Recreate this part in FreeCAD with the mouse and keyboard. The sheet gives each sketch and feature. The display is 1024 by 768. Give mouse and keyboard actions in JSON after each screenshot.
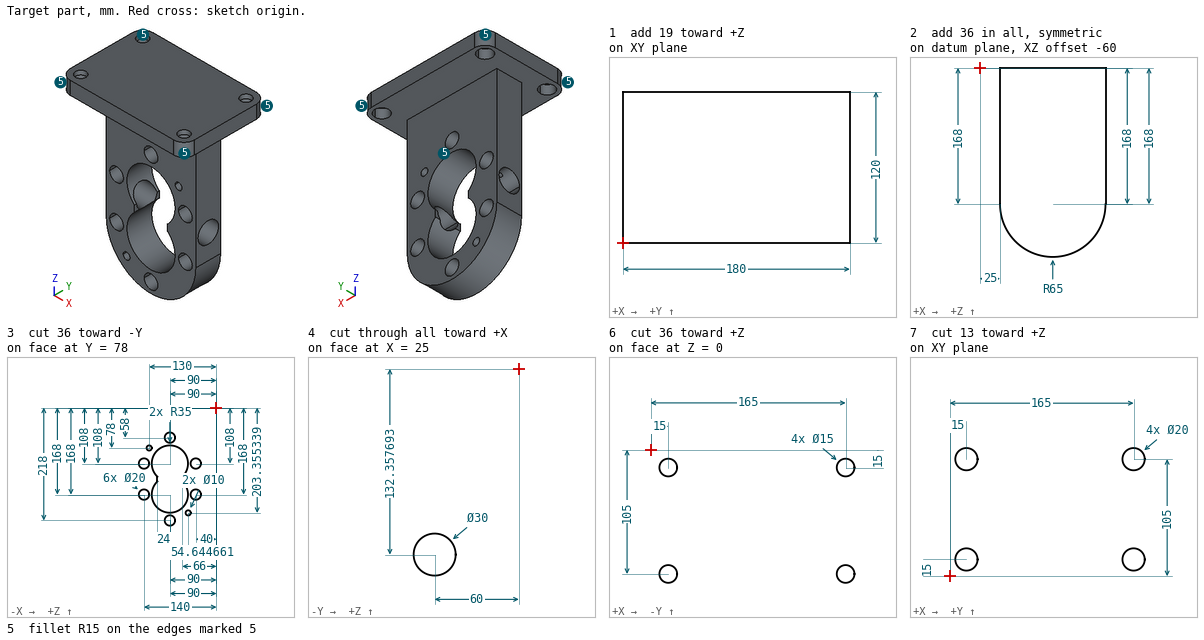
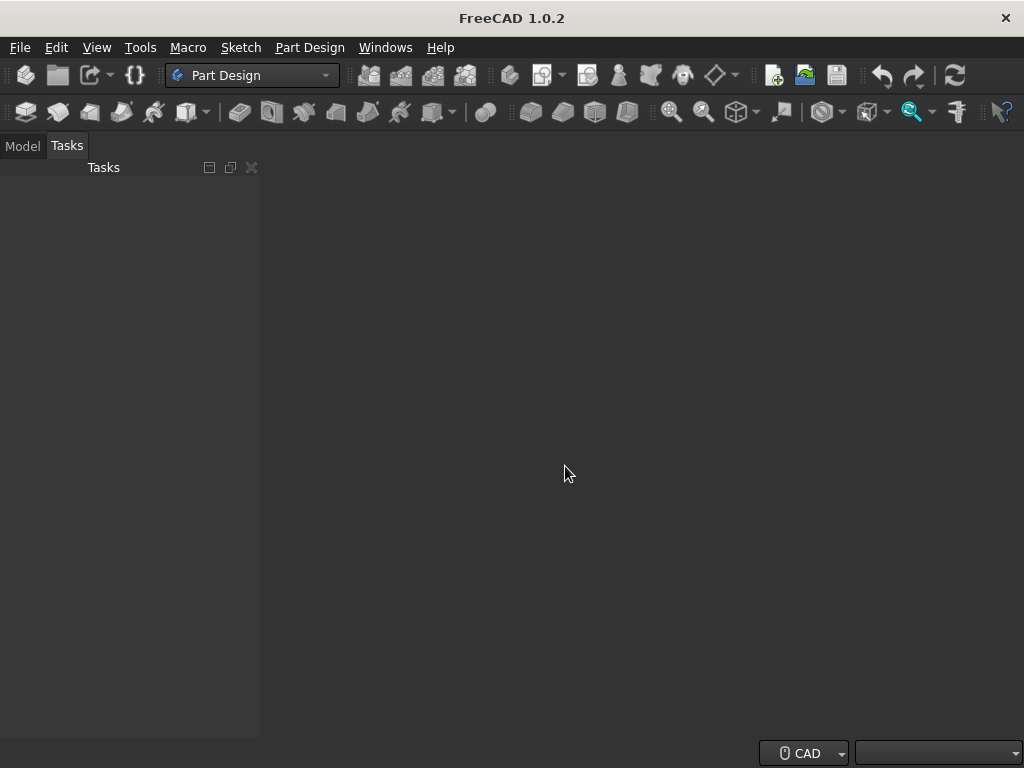
{"action": "left_click", "coordinate": [774, 76]}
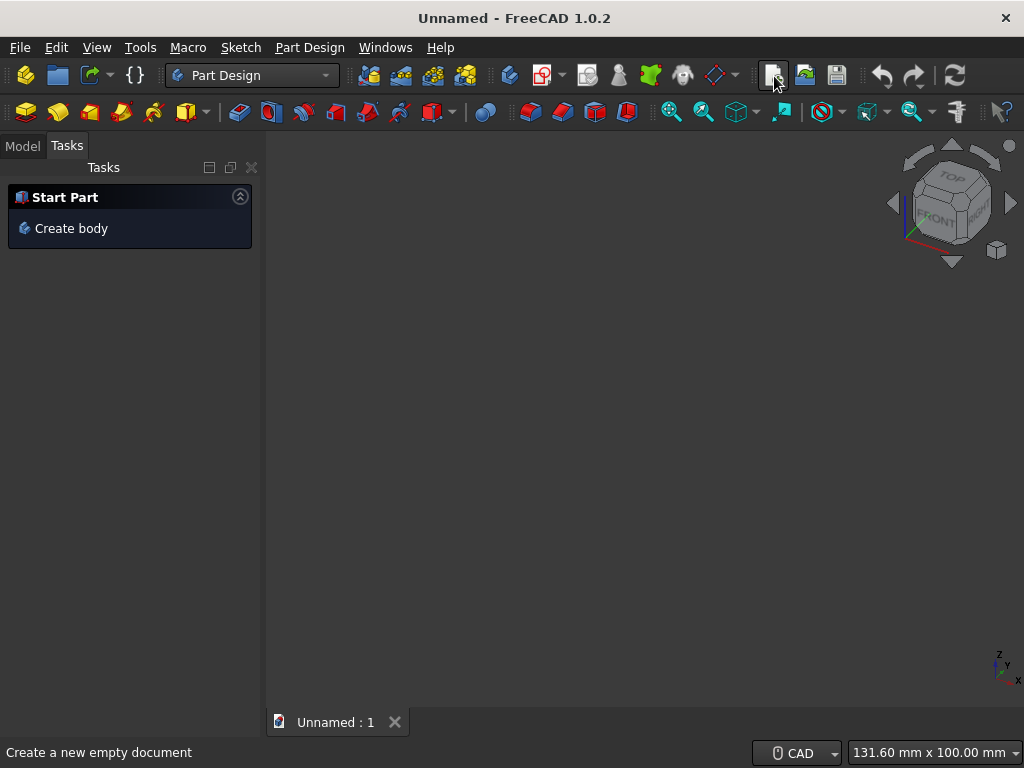
{"action": "left_click", "coordinate": [542, 76]}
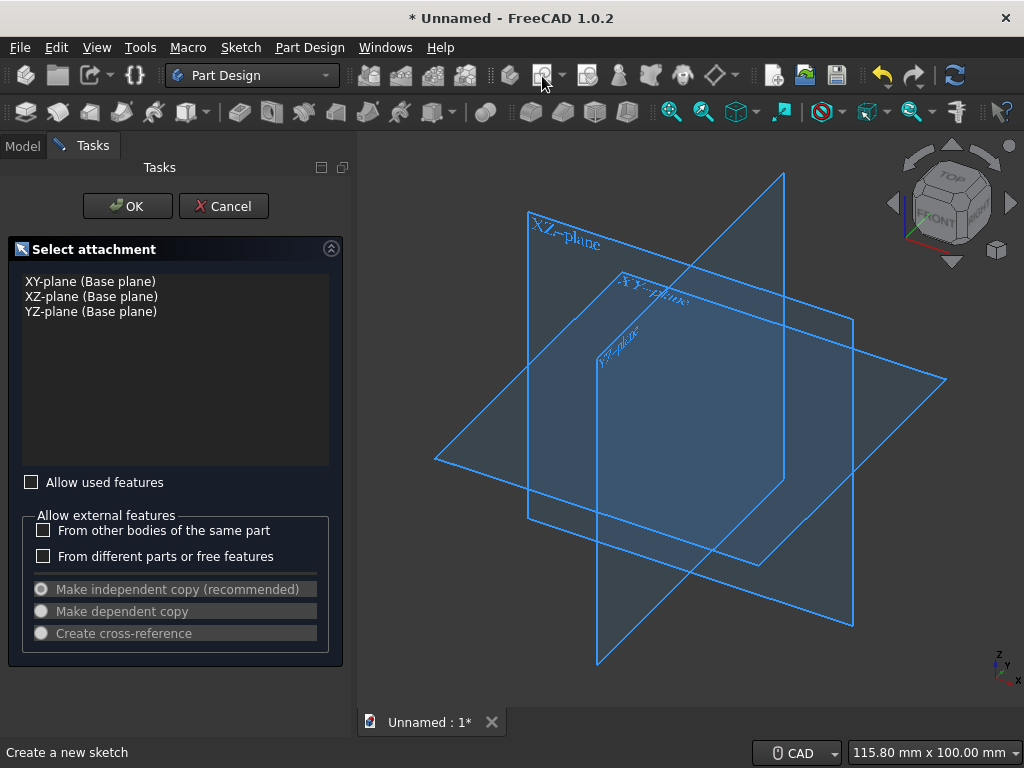
{"action": "left_click", "coordinate": [82, 282]}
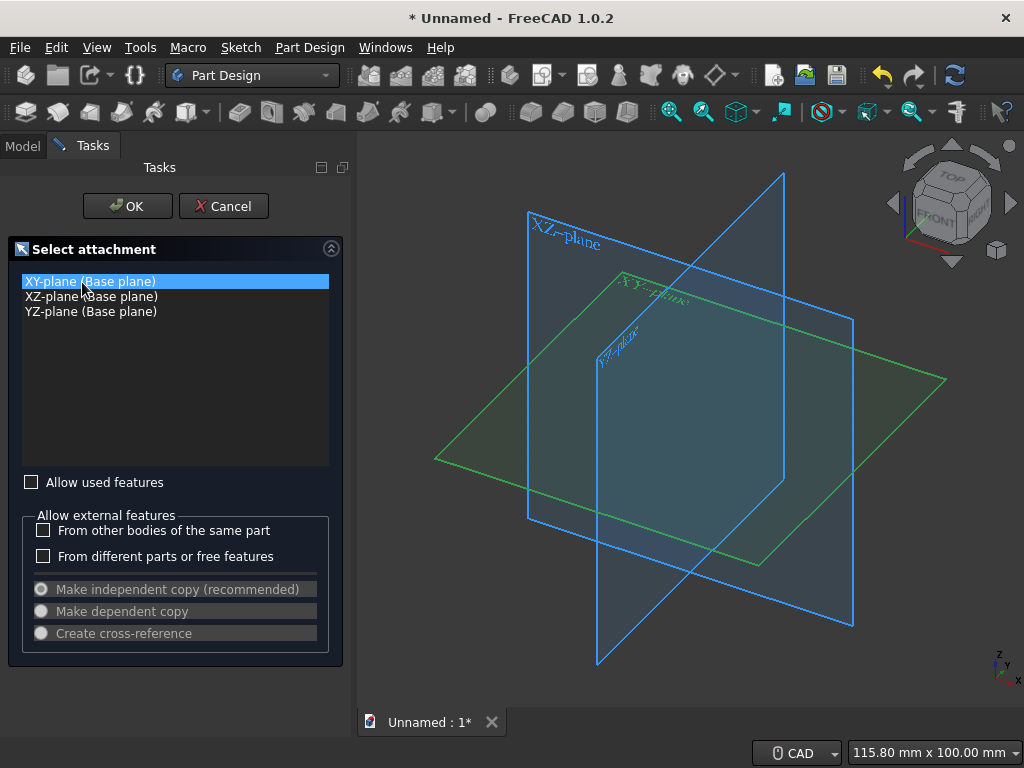
{"action": "left_click", "coordinate": [128, 206]}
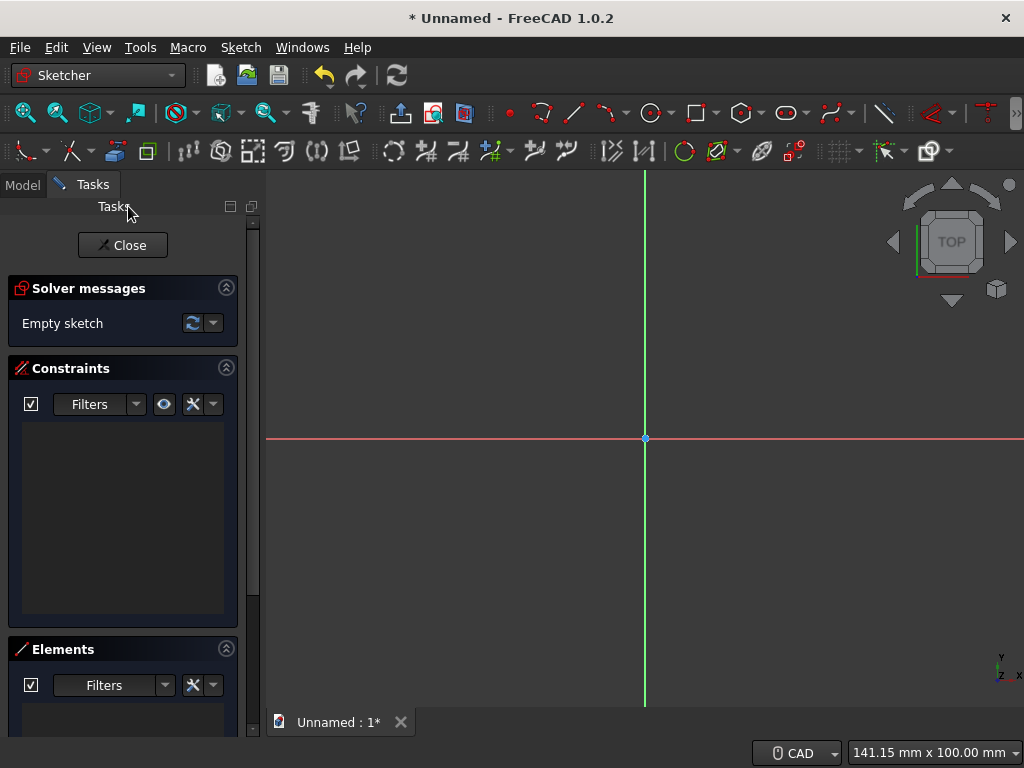
{"action": "scroll", "coordinate": [294, 626], "scroll_direction": "down", "scroll_amount": 5}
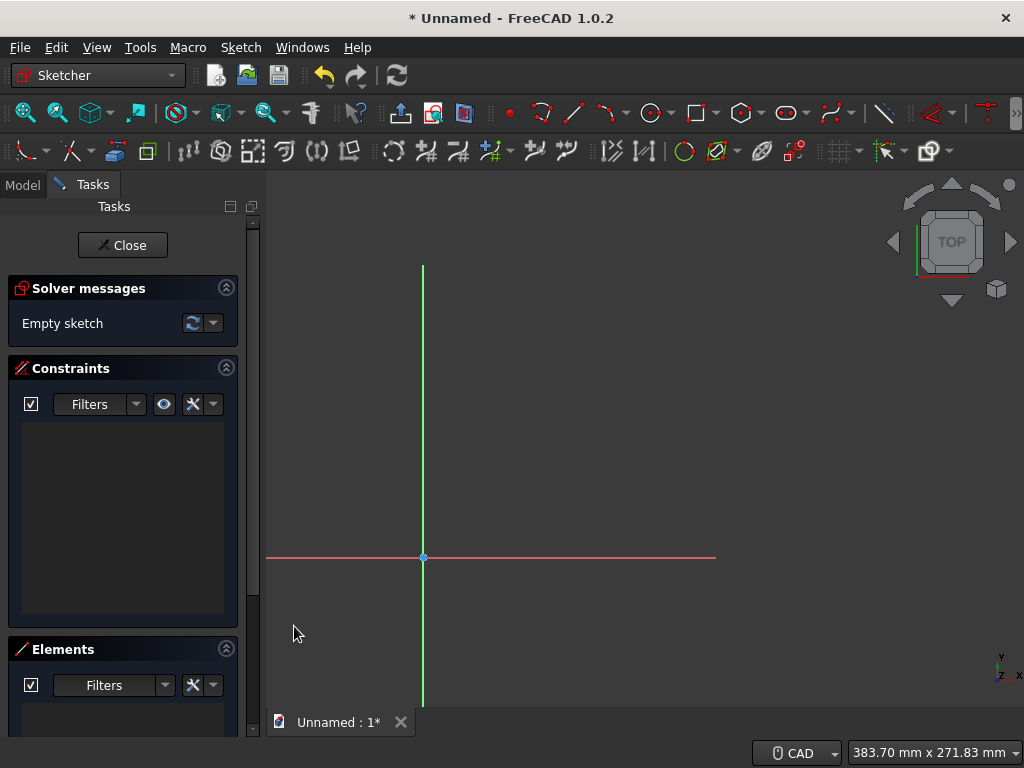
{"action": "left_click", "coordinate": [696, 114]}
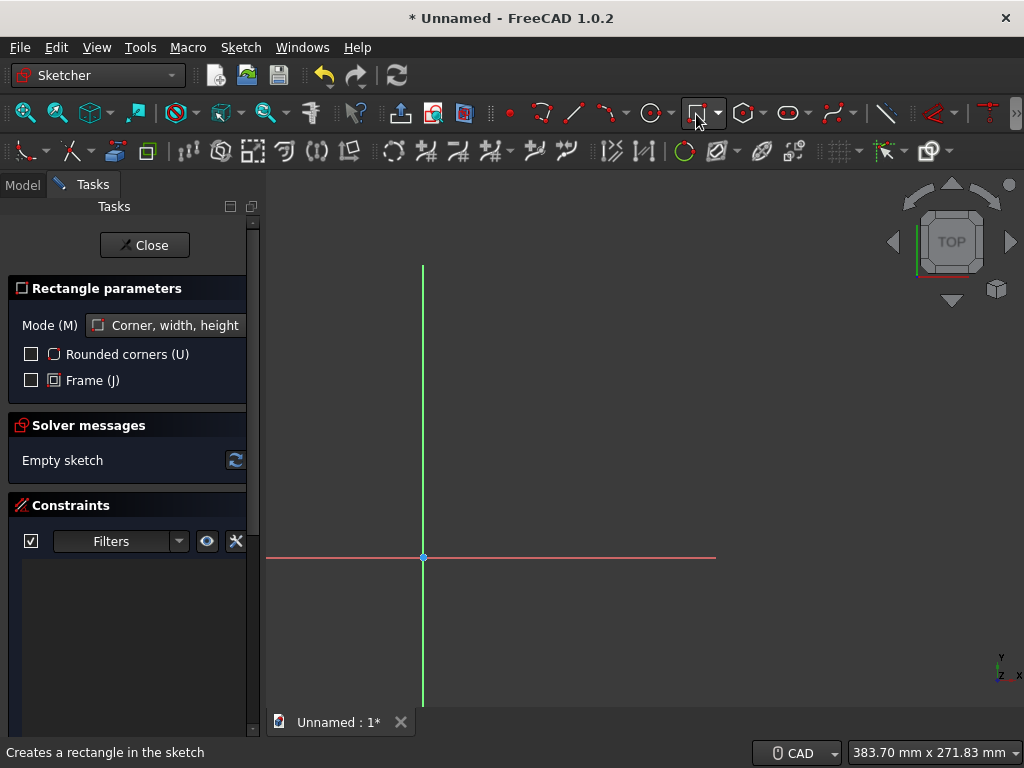
{"action": "left_click", "coordinate": [423, 558]}
{"action": "left_click", "coordinate": [779, 320]}
{"action": "key", "text": "Escape"}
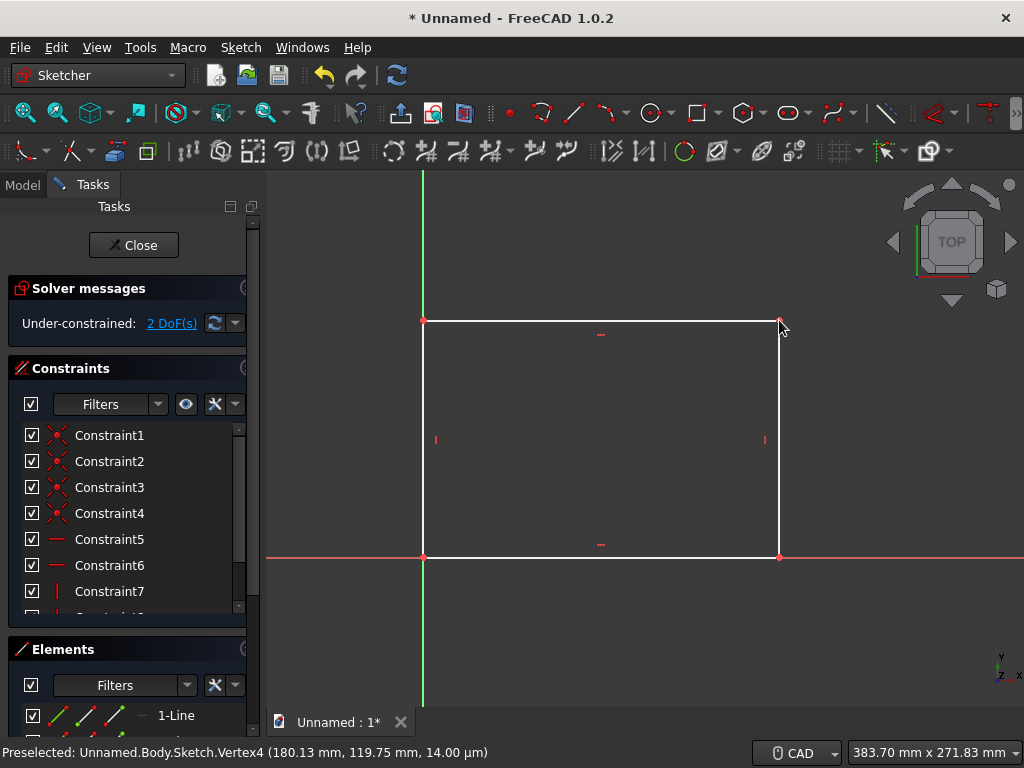
{"action": "left_click", "coordinate": [530, 558]}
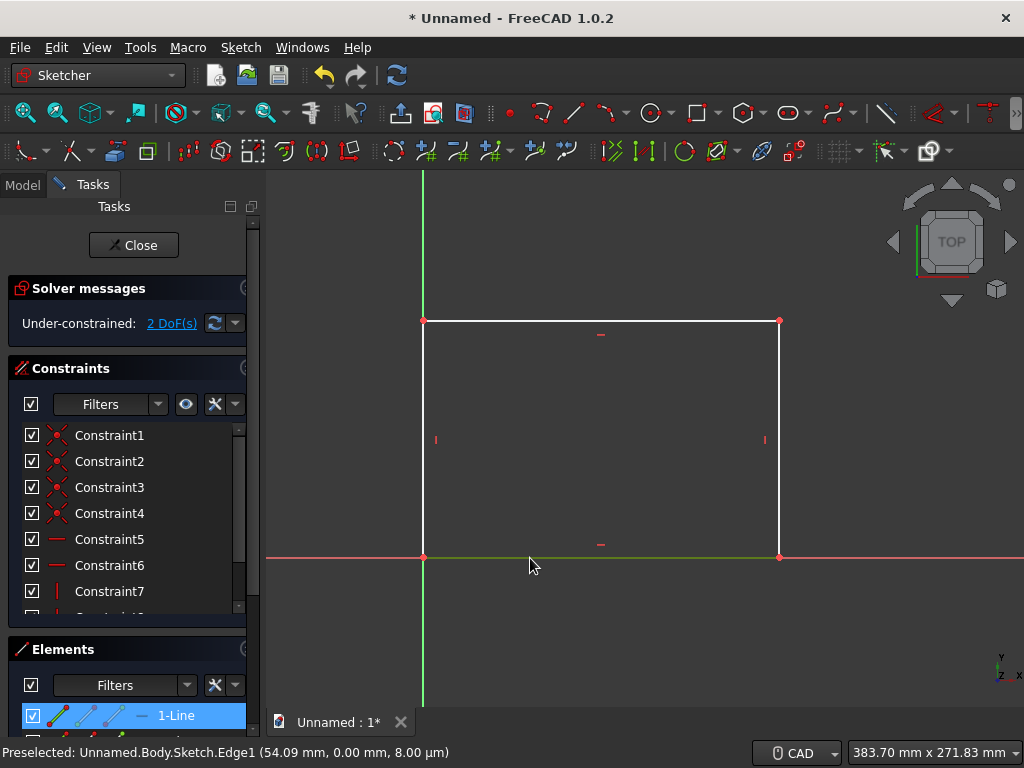
{"action": "left_click", "coordinate": [956, 114]}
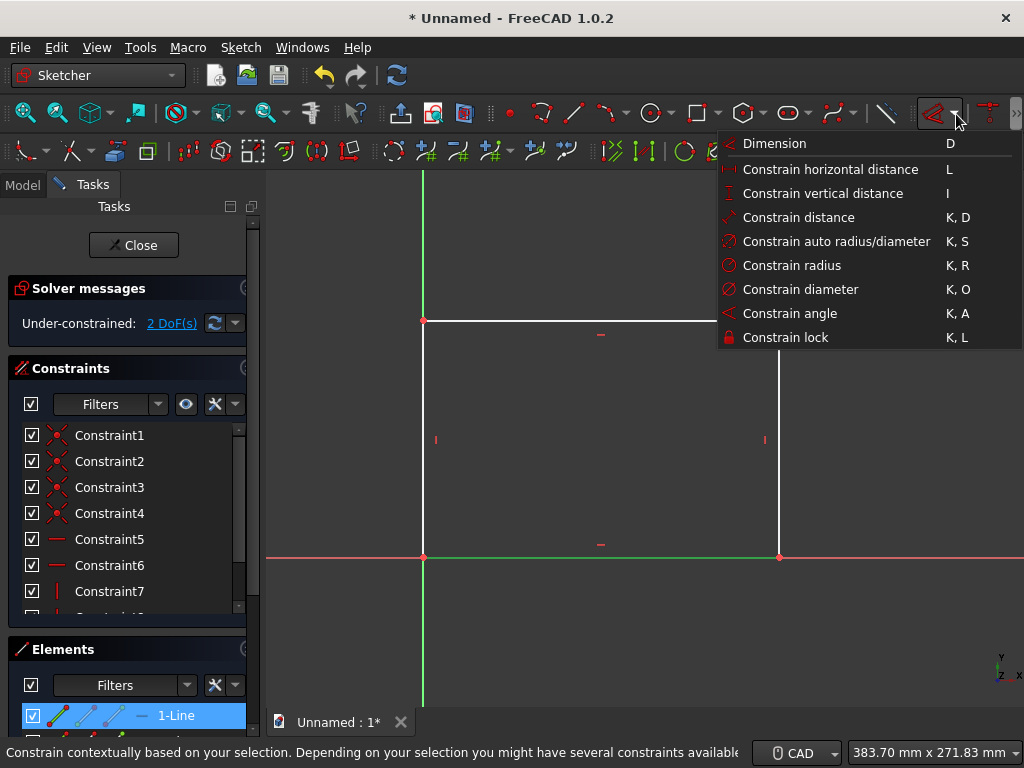
{"action": "left_click", "coordinate": [870, 169]}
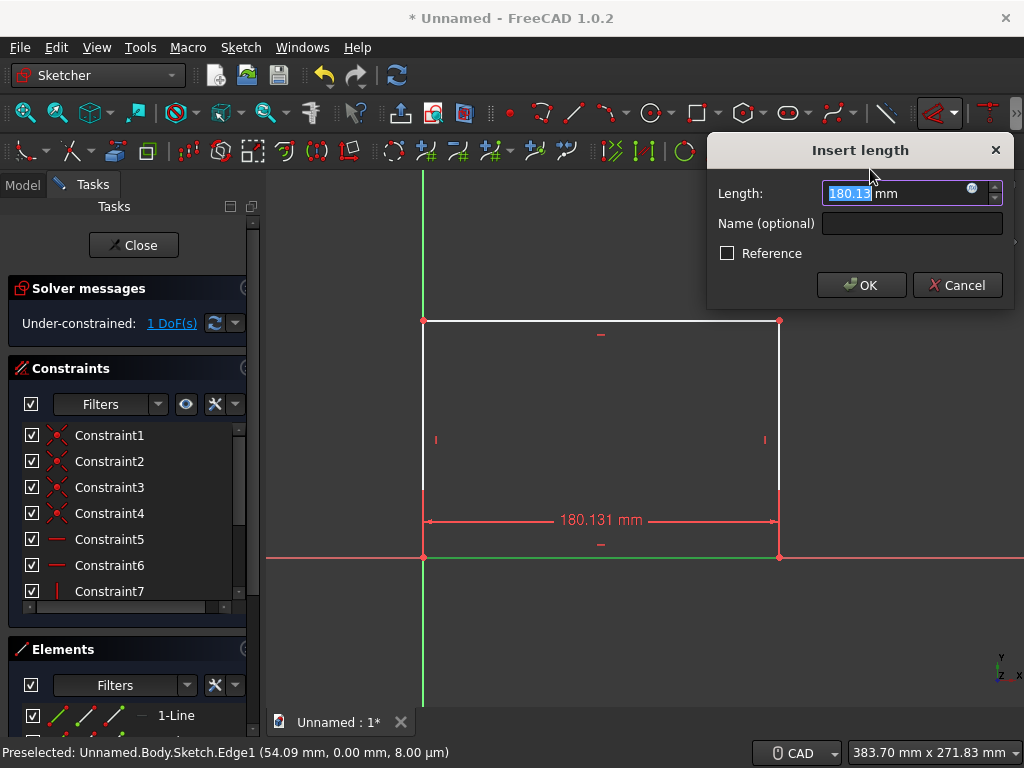
{"action": "type", "text": "180"}
{"action": "key", "text": "Return"}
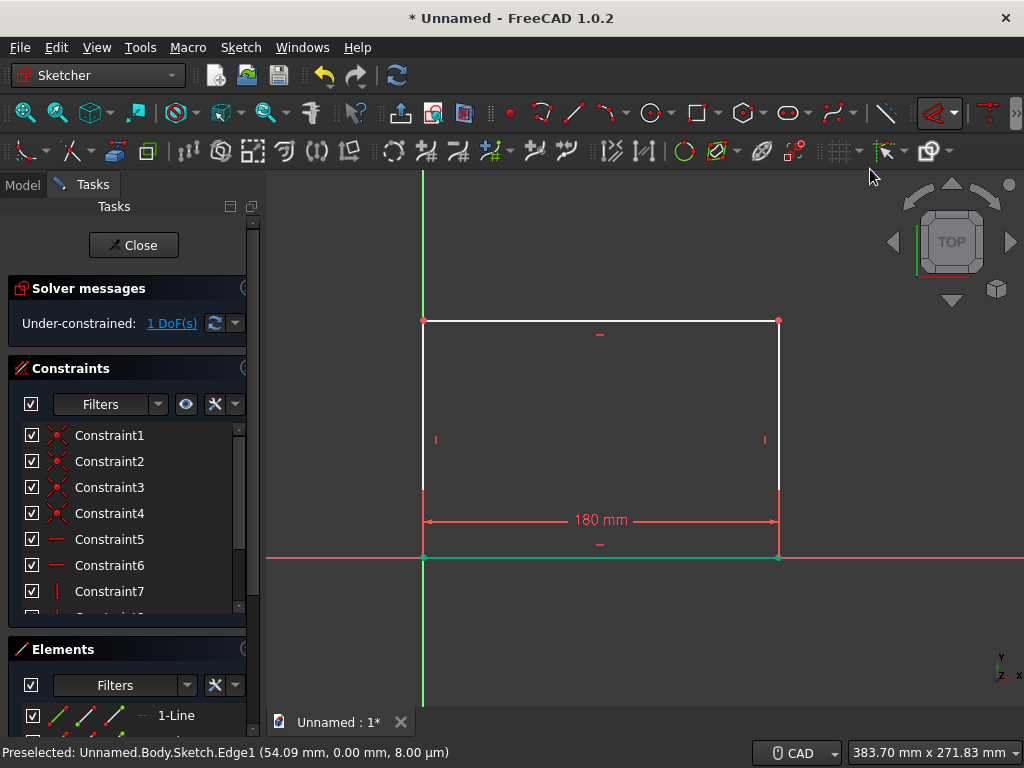
{"action": "left_click", "coordinate": [779, 487]}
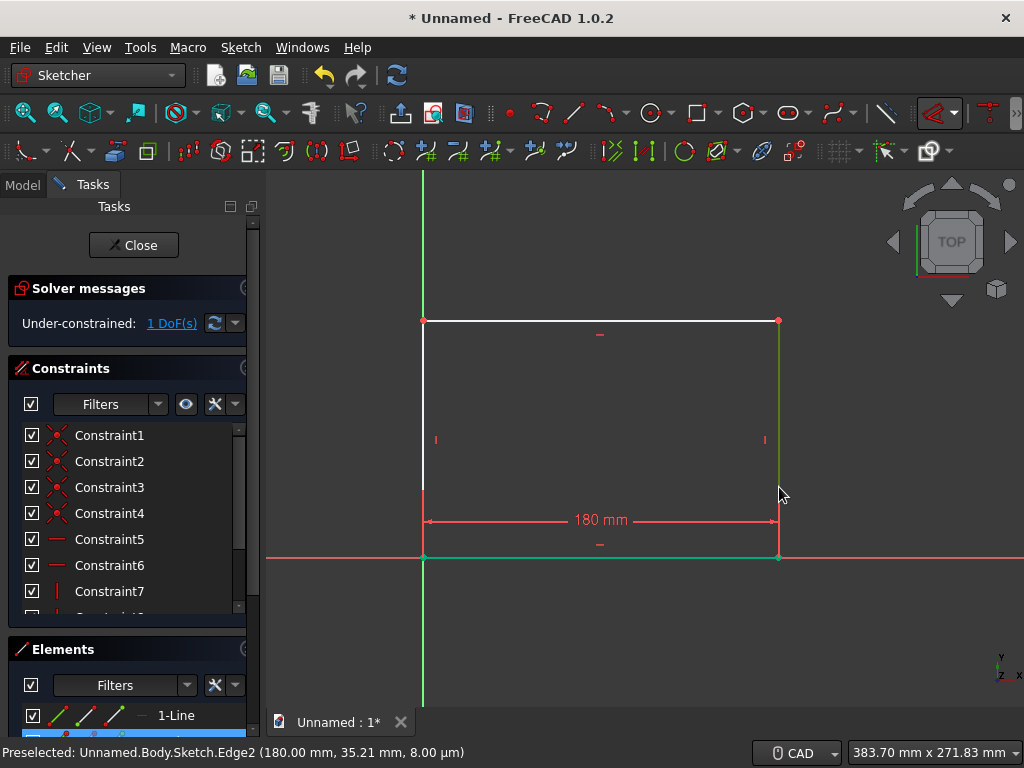
{"action": "key", "text": "i"}